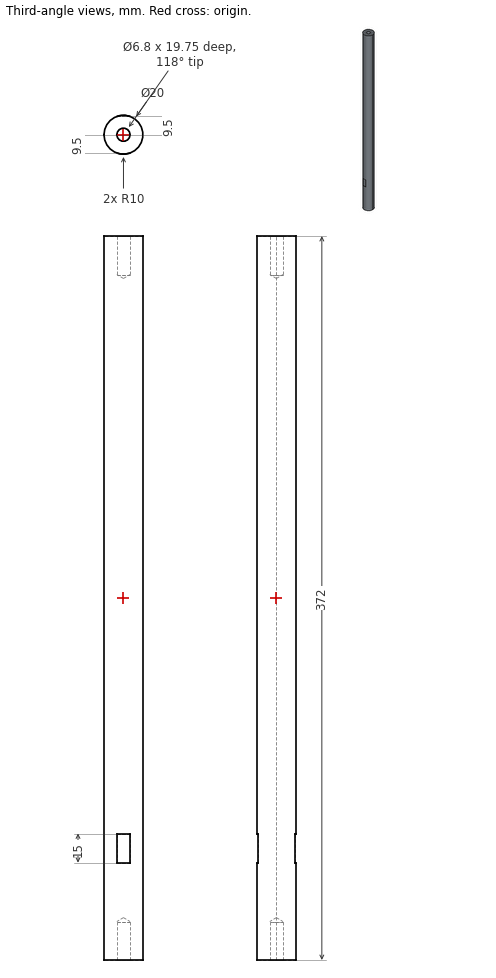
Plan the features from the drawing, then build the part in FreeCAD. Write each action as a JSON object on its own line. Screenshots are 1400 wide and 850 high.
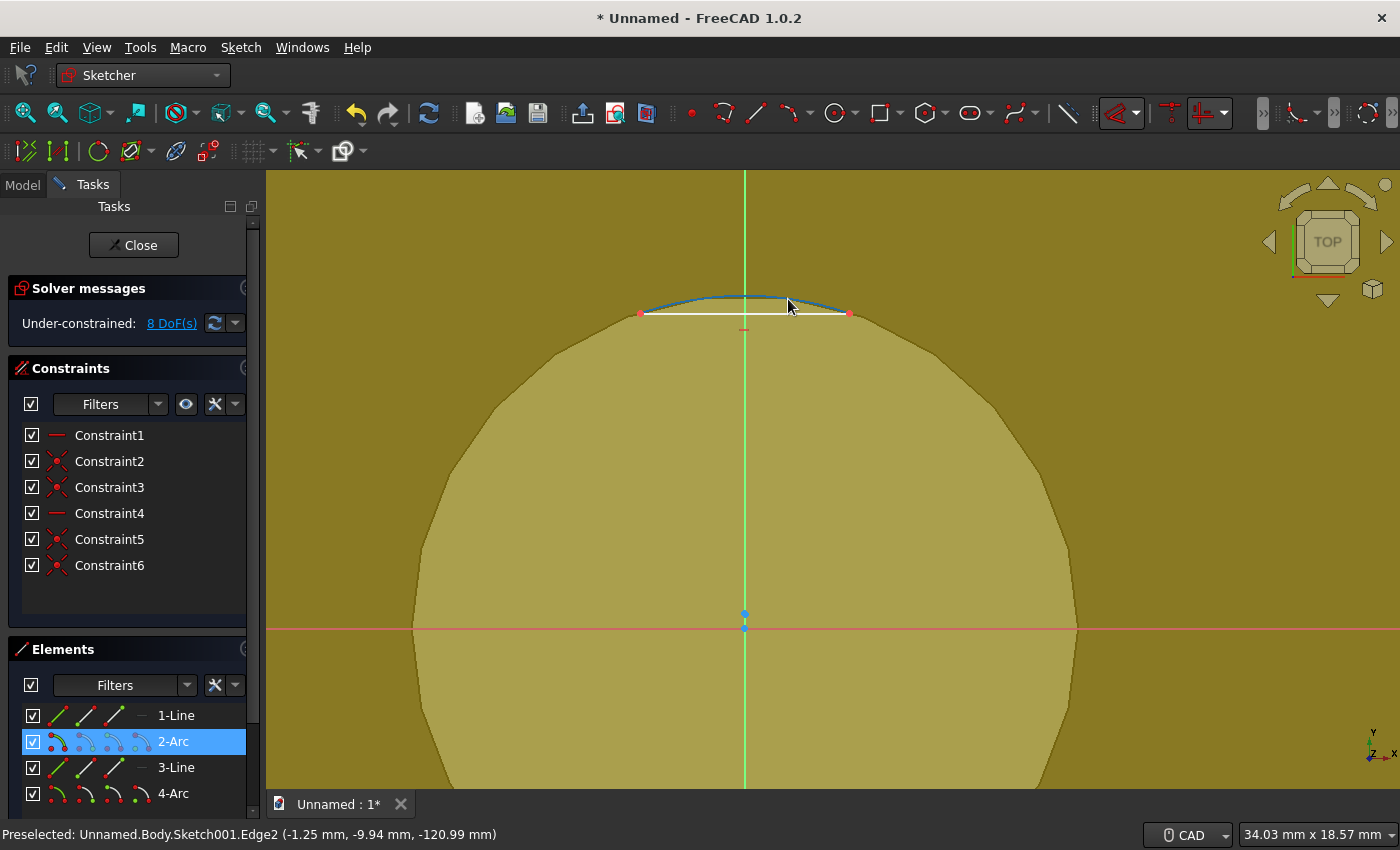
{"action": "left_click", "coordinate": [787, 299]}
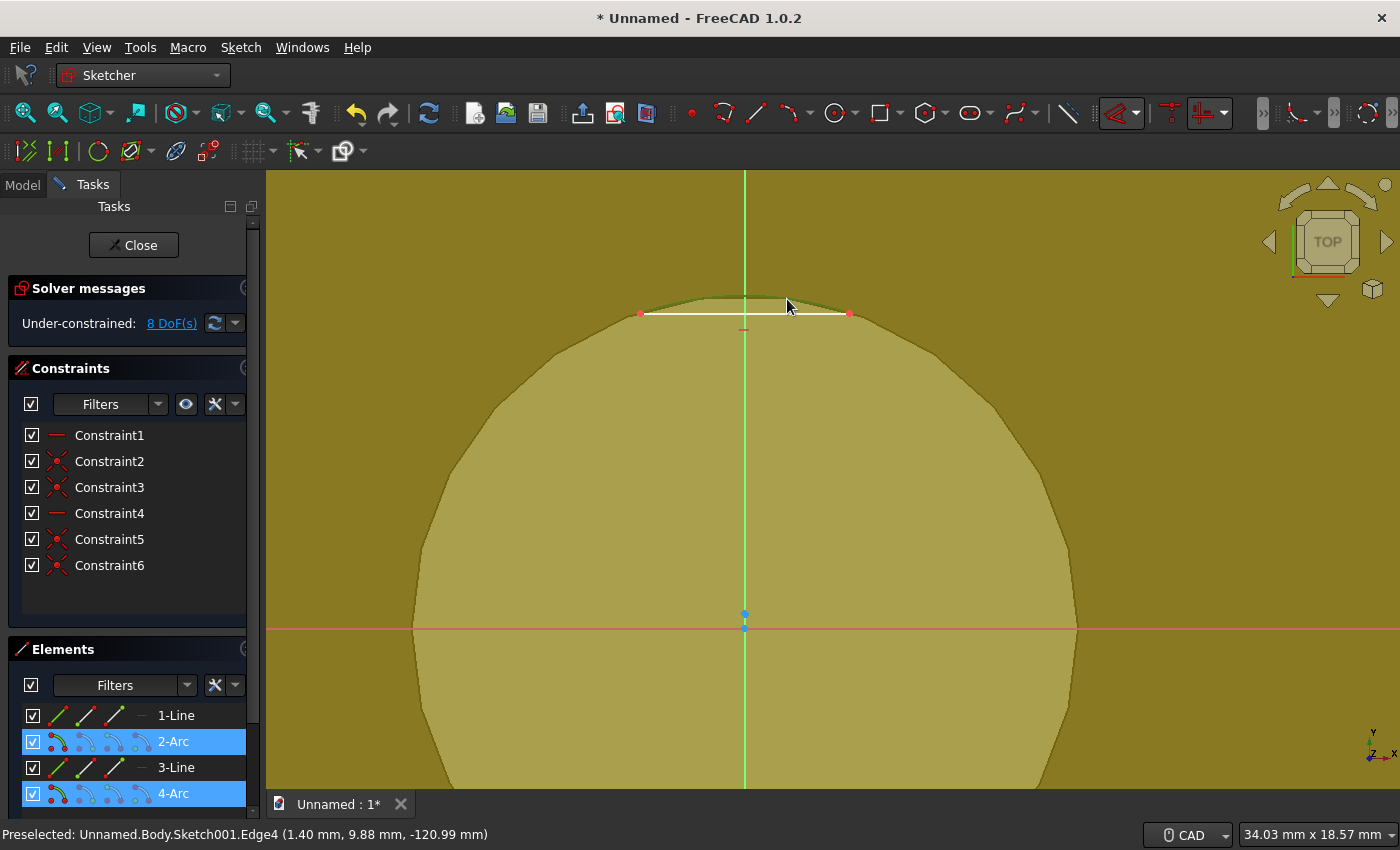
{"action": "left_click", "coordinate": [1170, 114]}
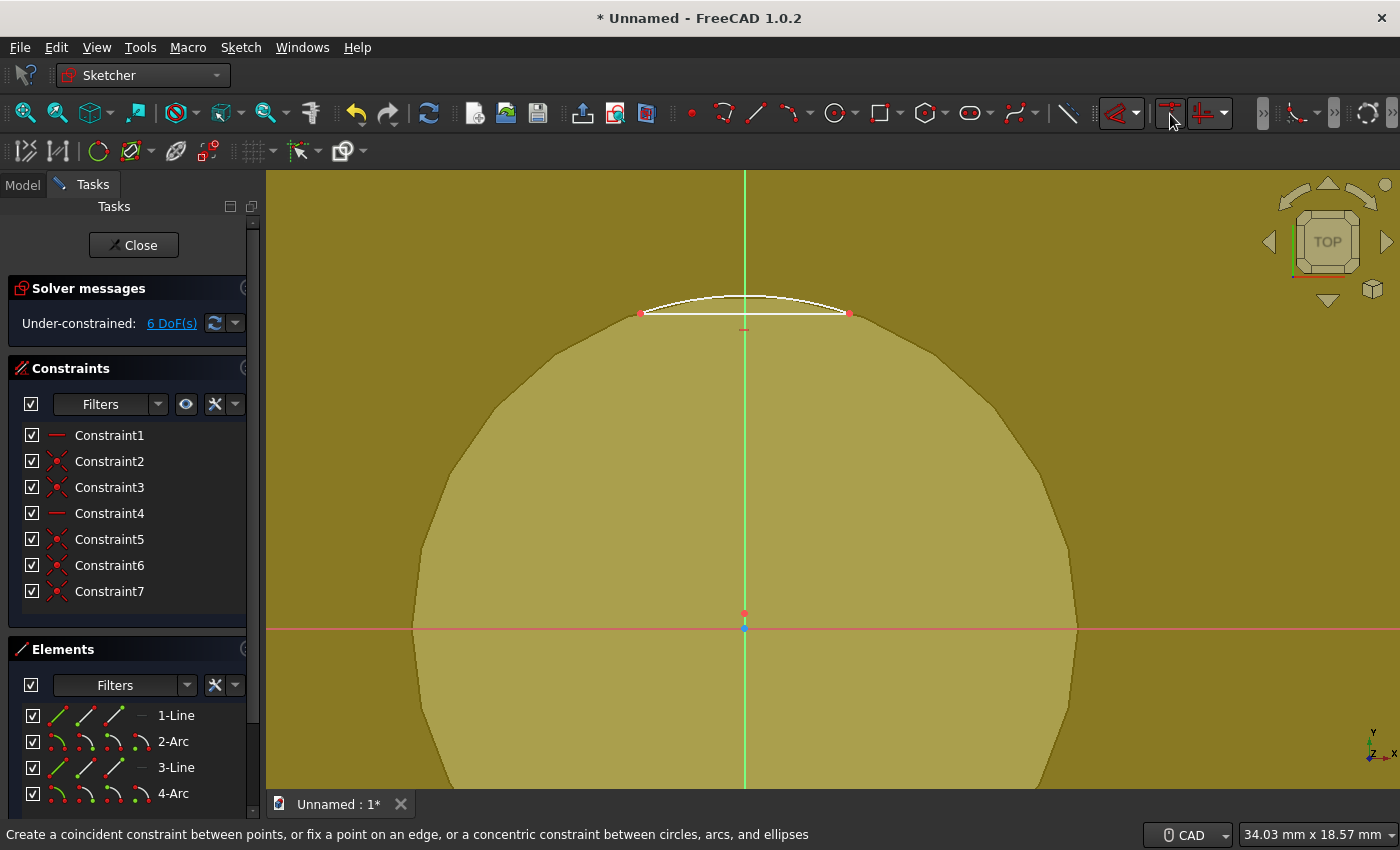
{"action": "left_click_drag", "start_coordinate": [735, 604], "coordinate": [755, 639]}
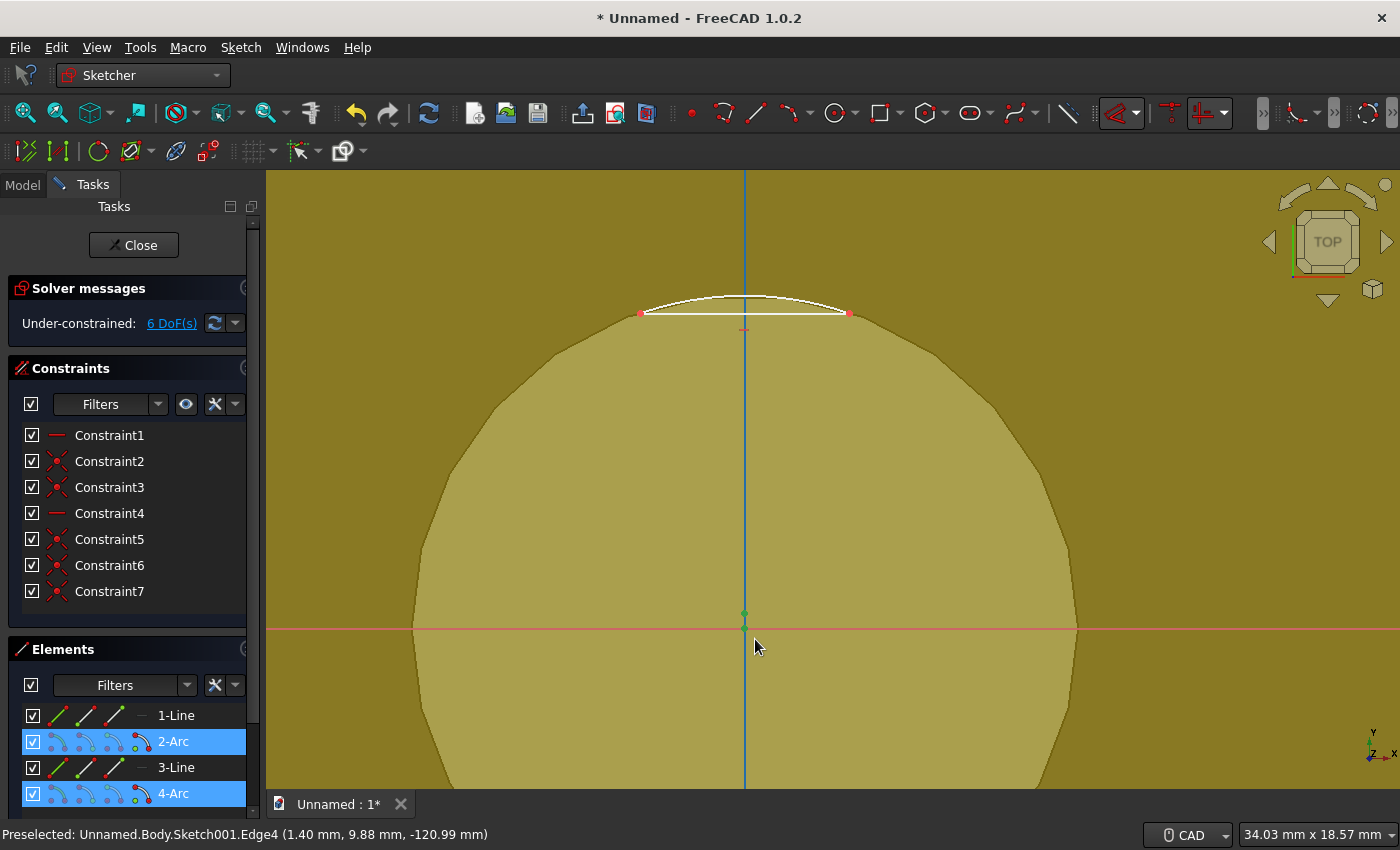
{"action": "left_click", "coordinate": [1170, 114]}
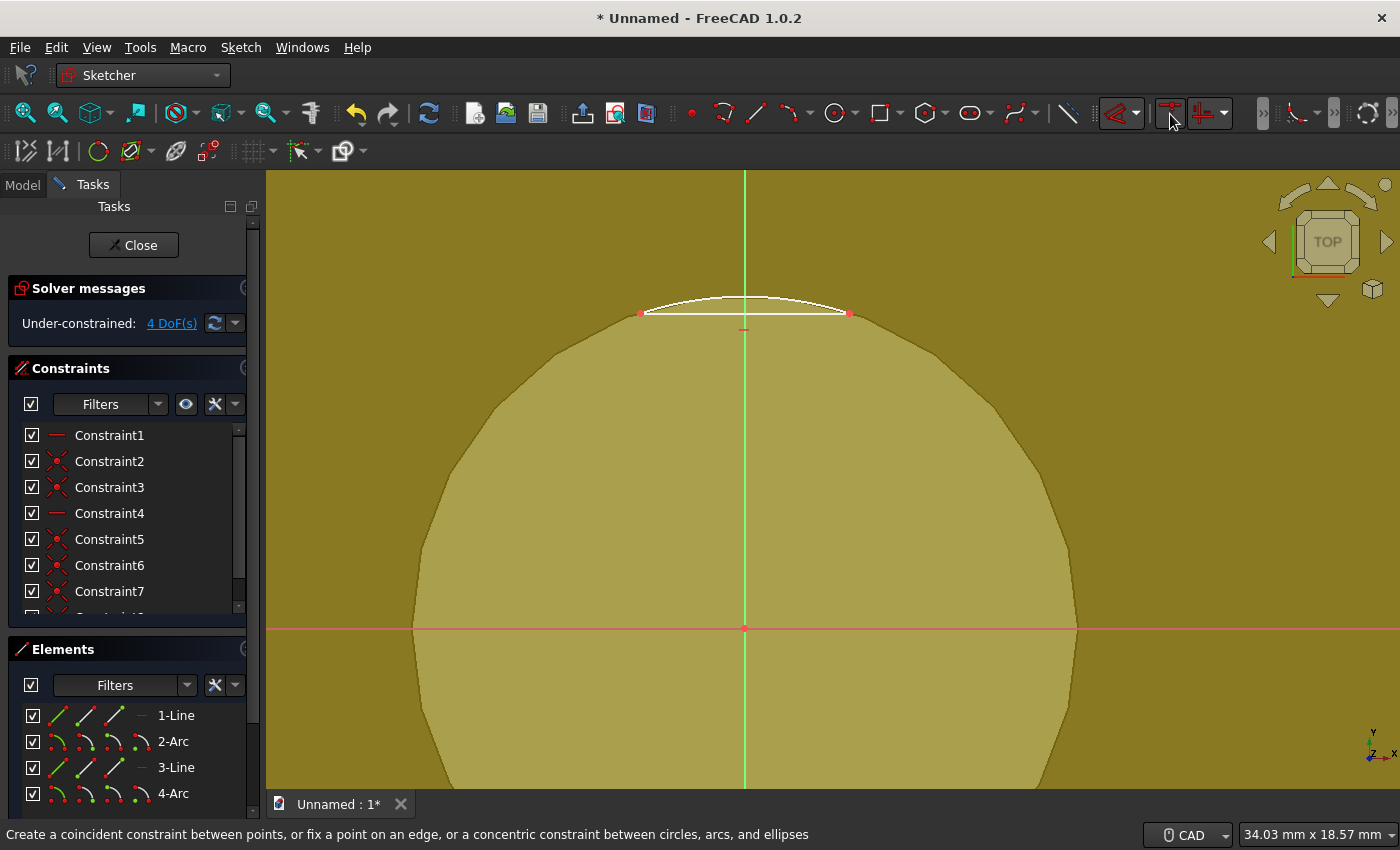
{"action": "scroll", "coordinate": [788, 298], "scroll_direction": "down", "scroll_amount": 3}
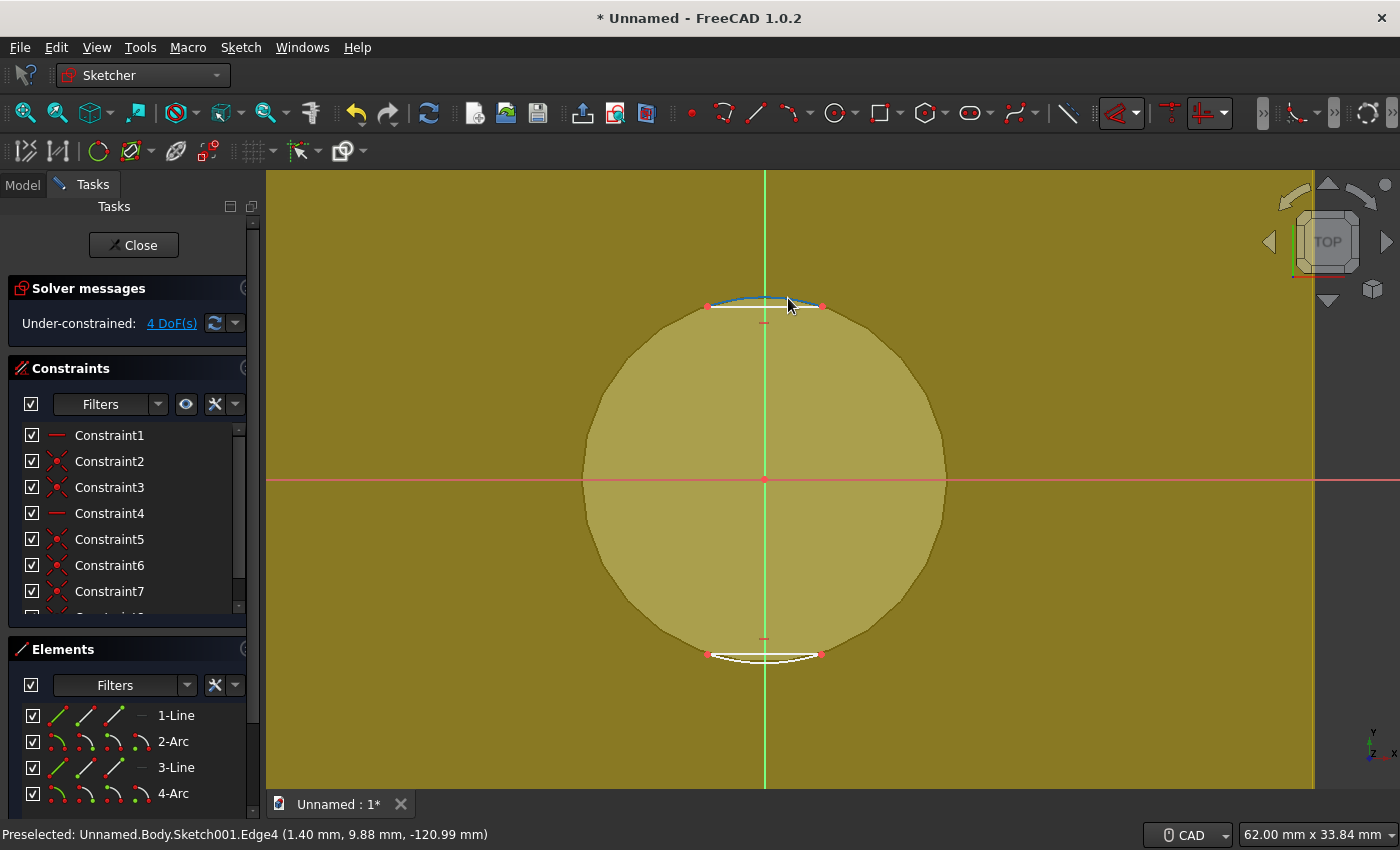
{"action": "scroll", "coordinate": [742, 662], "scroll_direction": "up", "scroll_amount": 4}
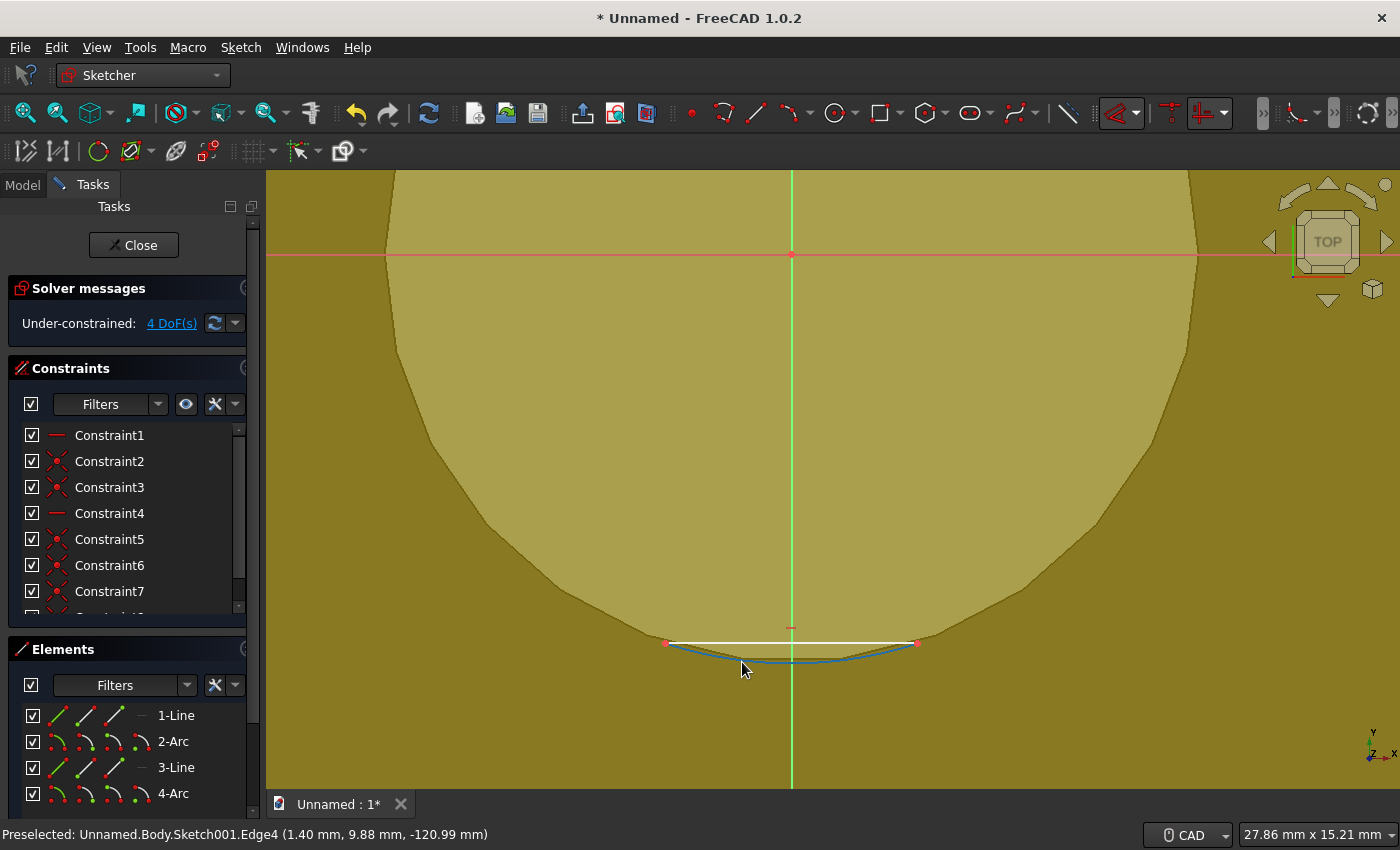
{"action": "left_click", "coordinate": [740, 660]}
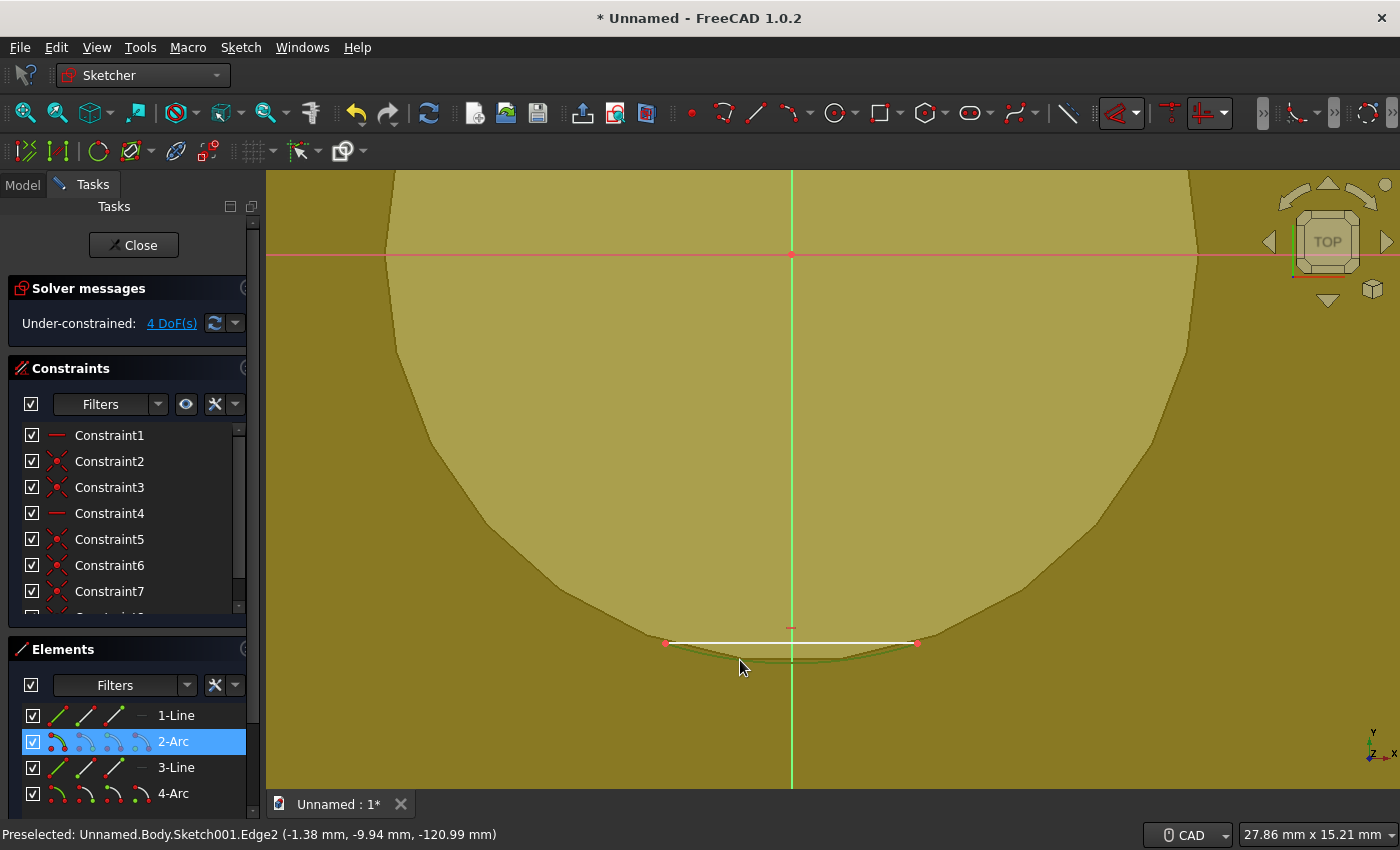
{"action": "scroll", "coordinate": [742, 663], "scroll_direction": "down", "scroll_amount": 4}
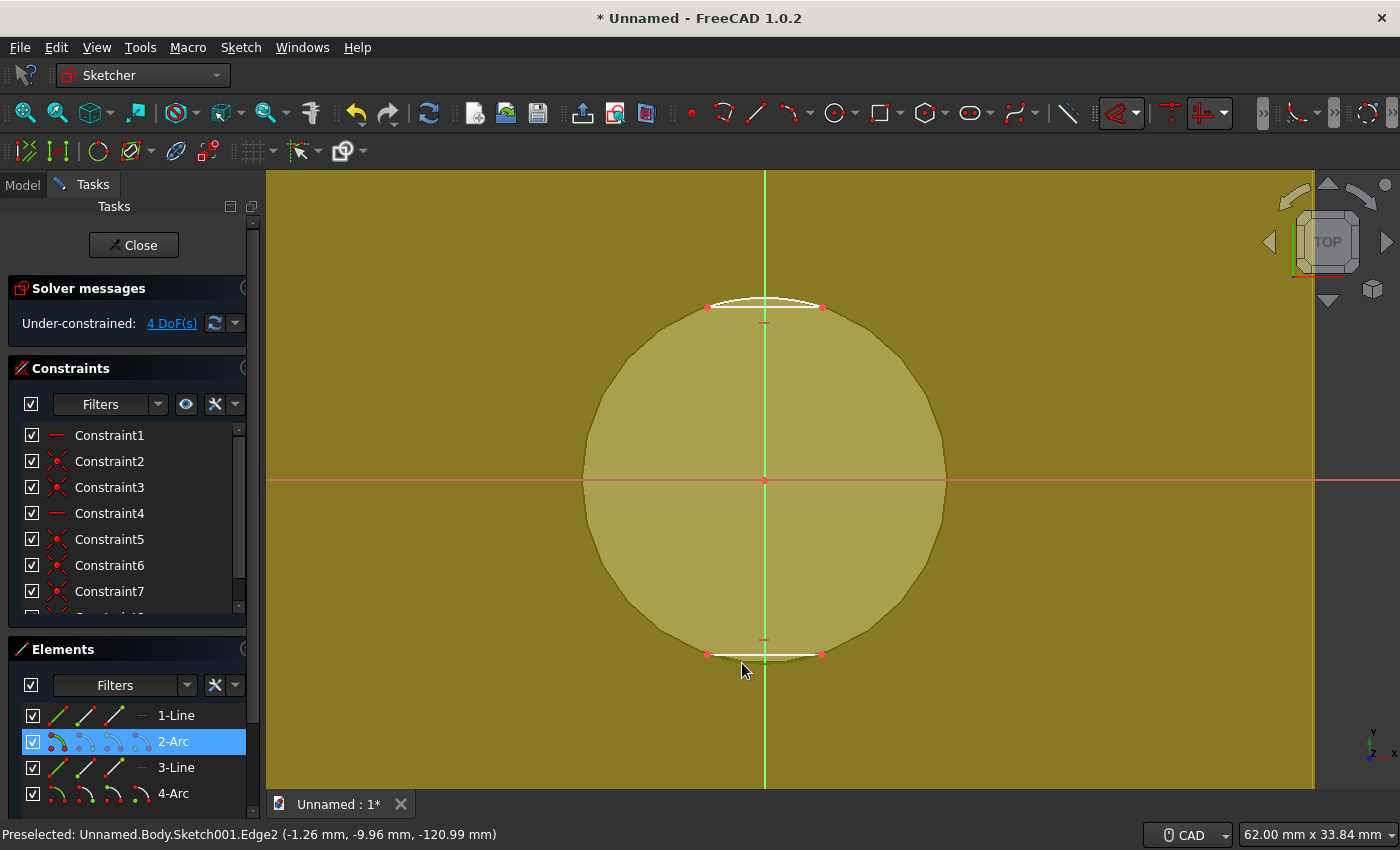
{"action": "scroll", "coordinate": [788, 299], "scroll_direction": "up", "scroll_amount": 3}